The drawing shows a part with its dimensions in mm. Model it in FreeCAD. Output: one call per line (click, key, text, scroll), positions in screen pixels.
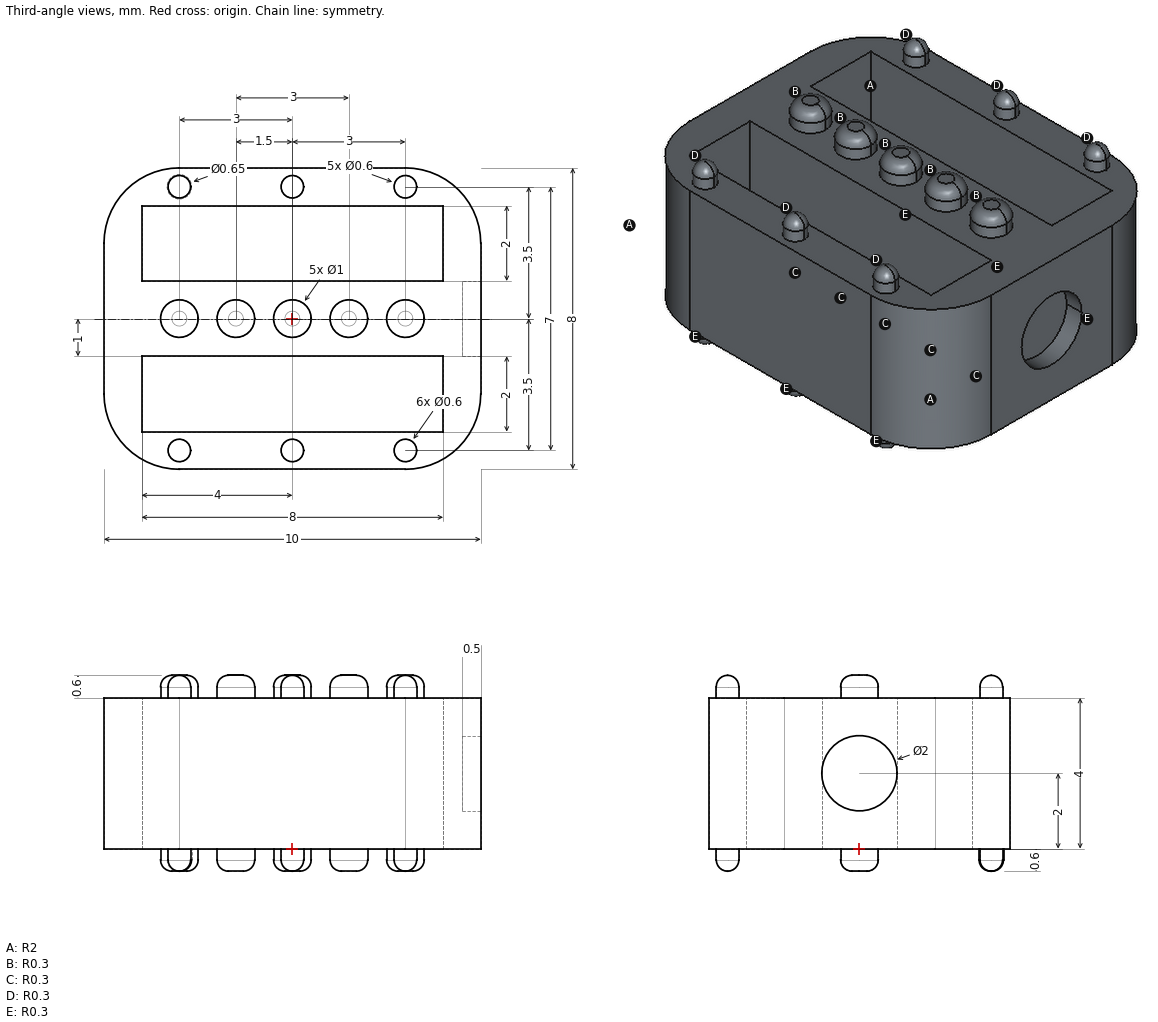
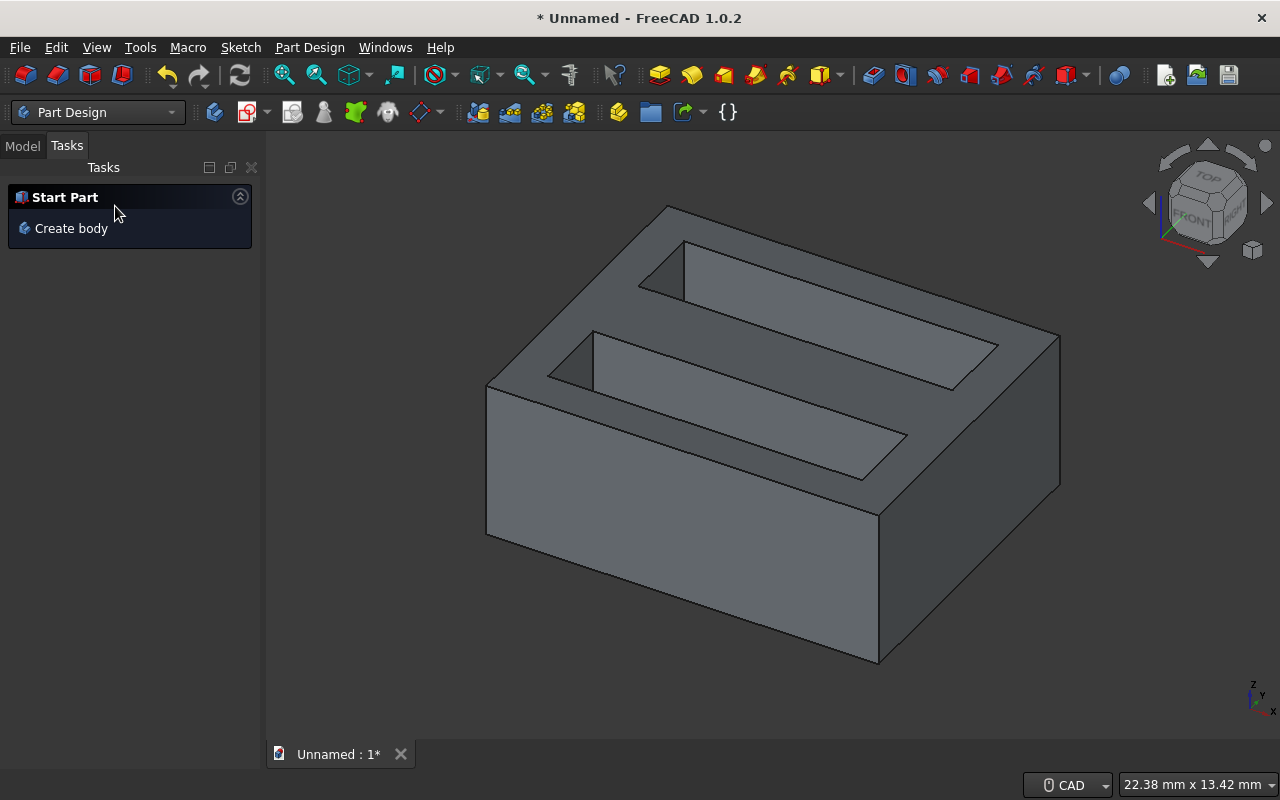
click(995, 473)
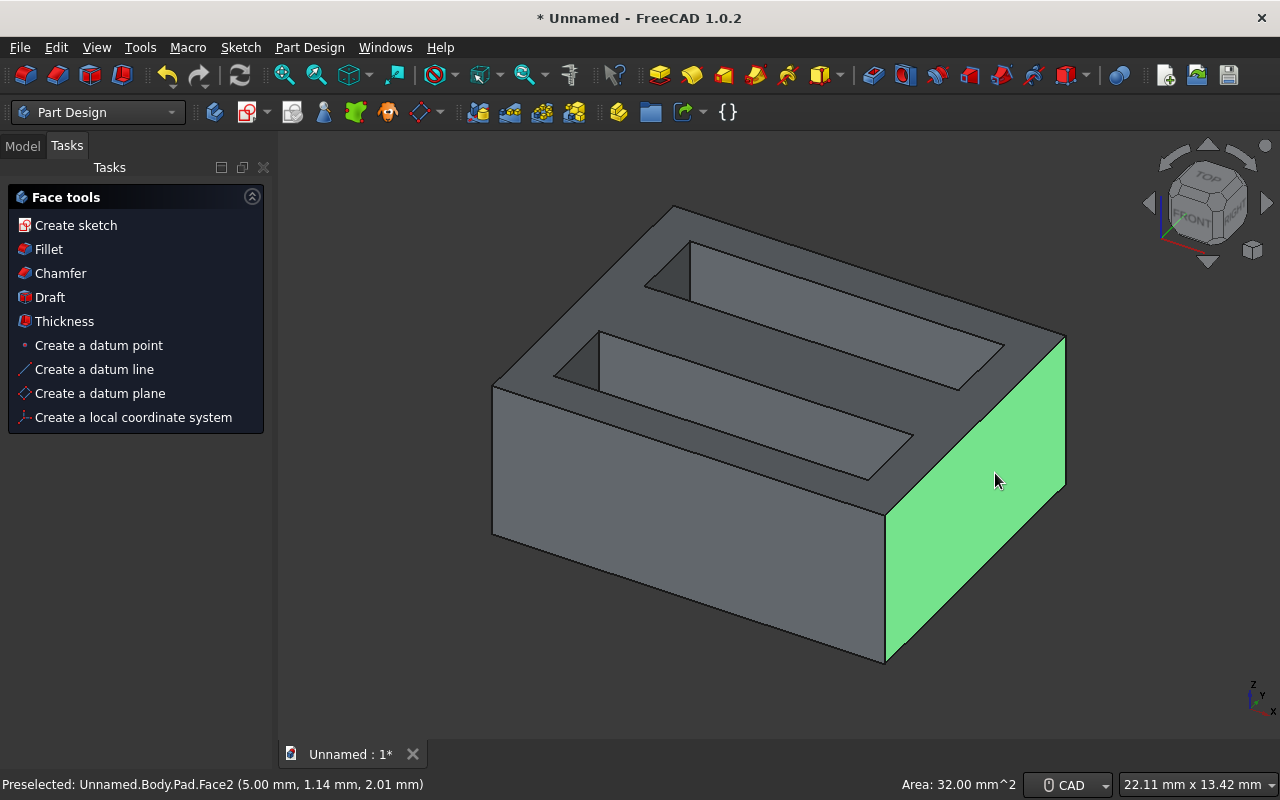
click(248, 112)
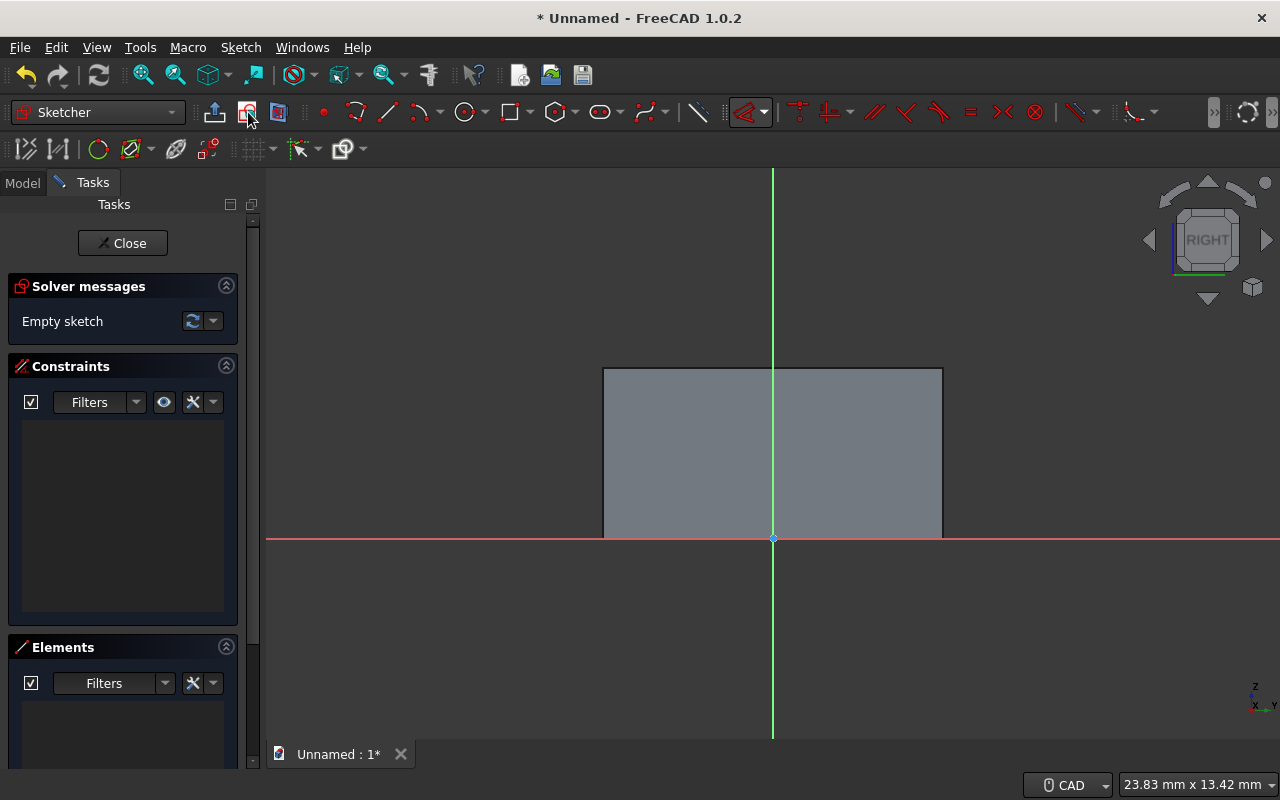
scroll(813, 487, up, 5)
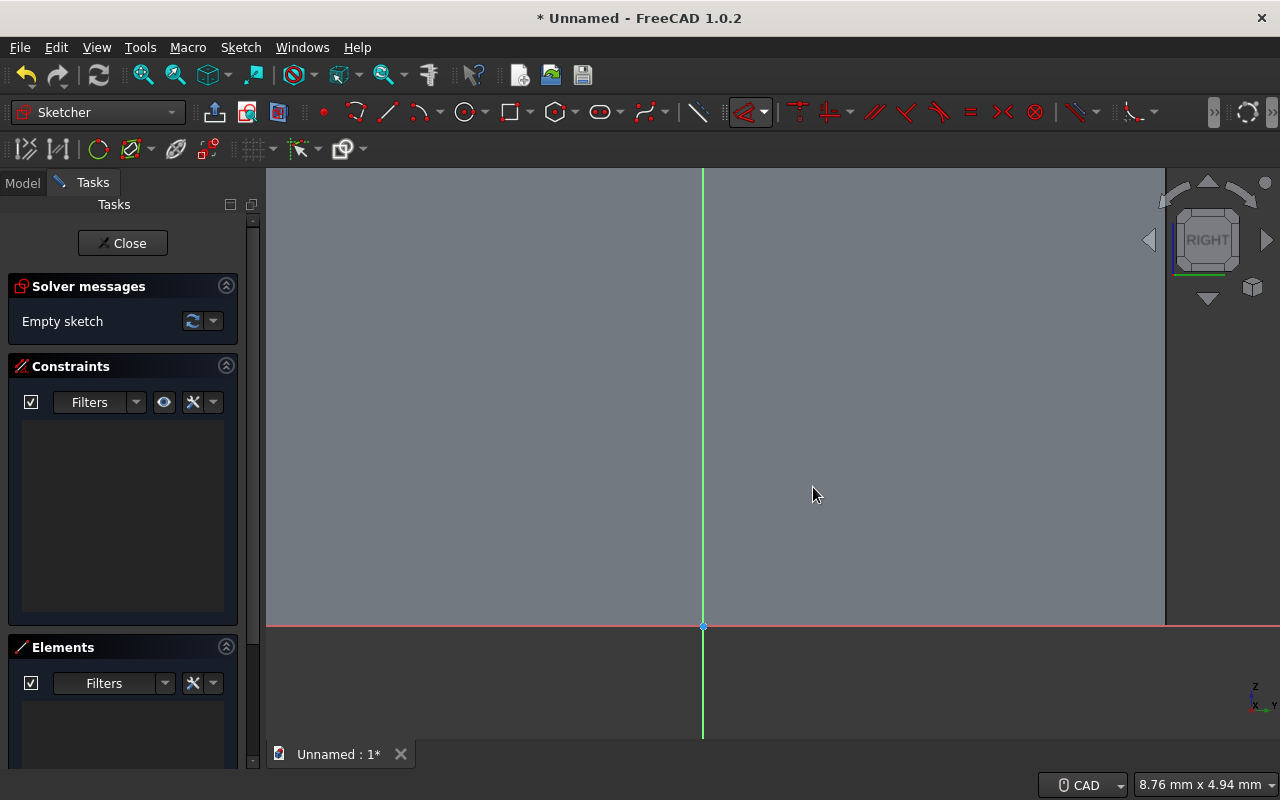
click(466, 112)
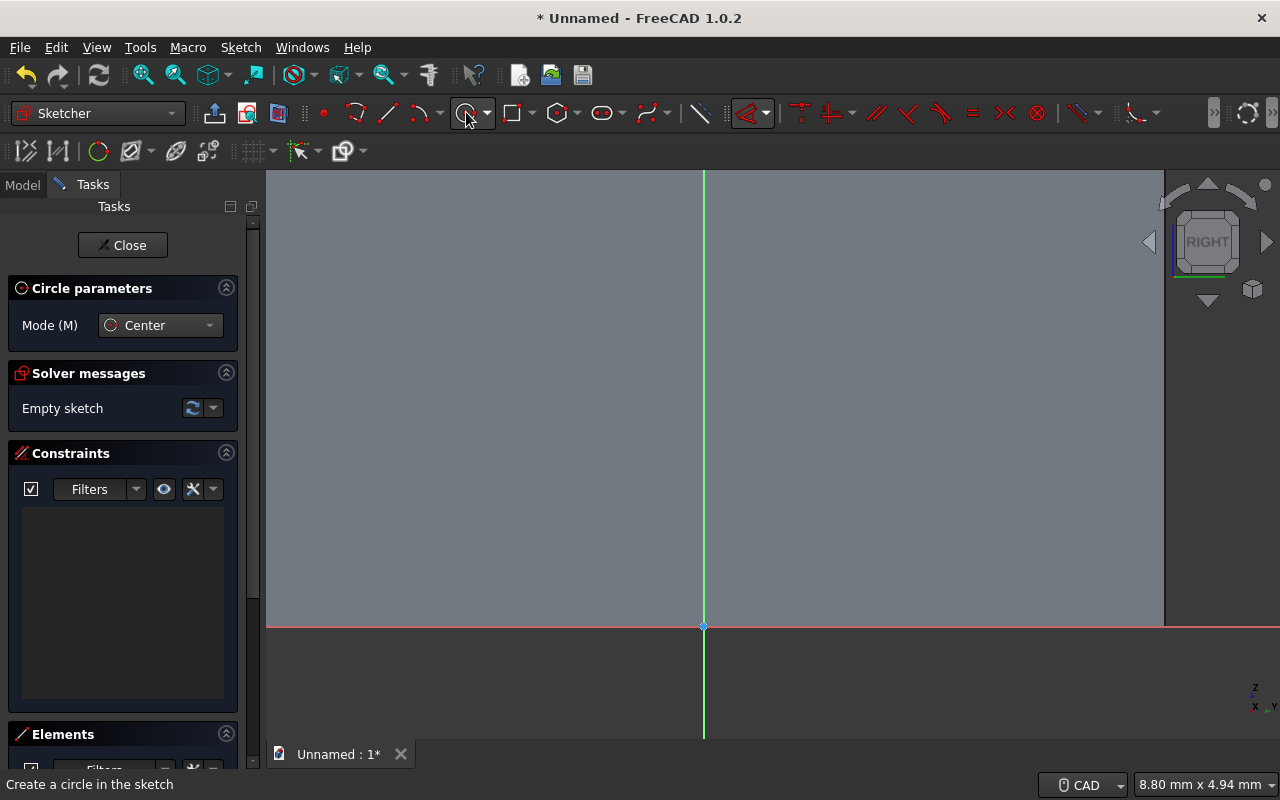
click(704, 396)
move(785, 315)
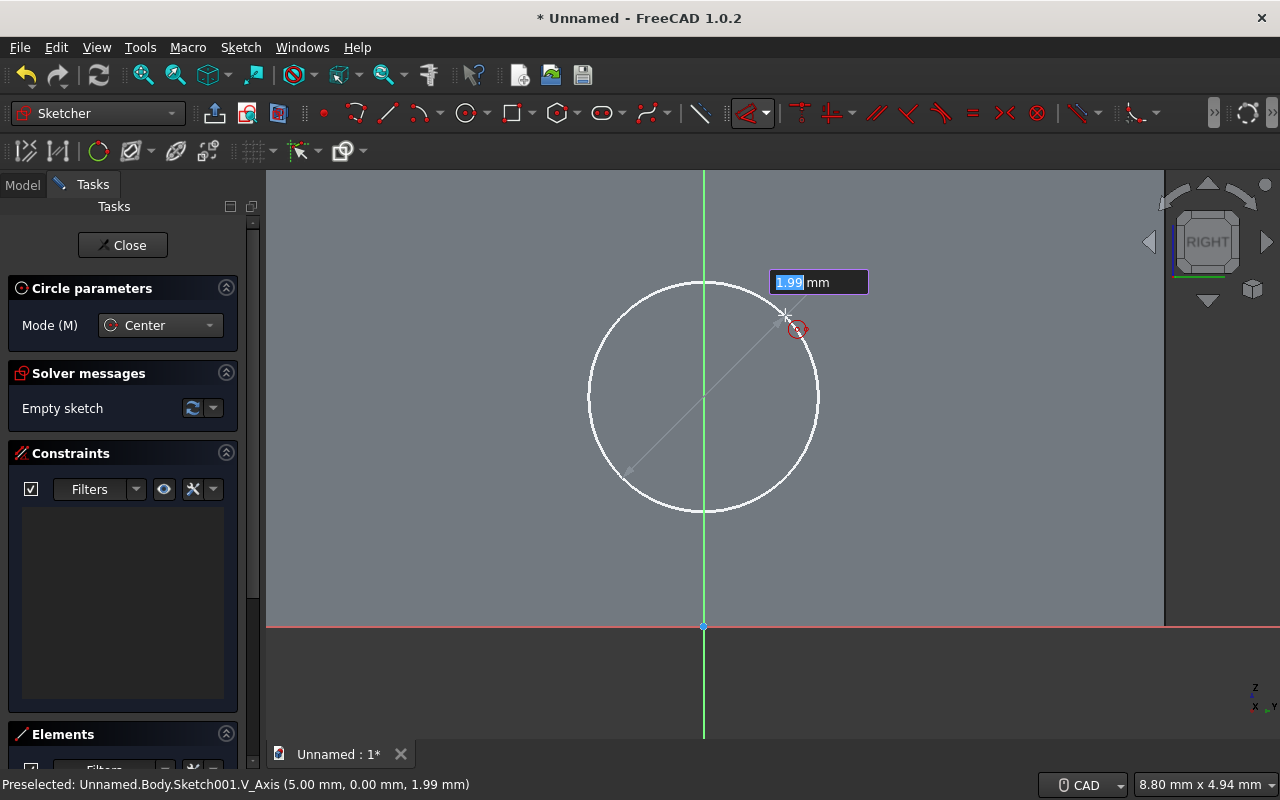
text(2)
key(Return)
key(Escape)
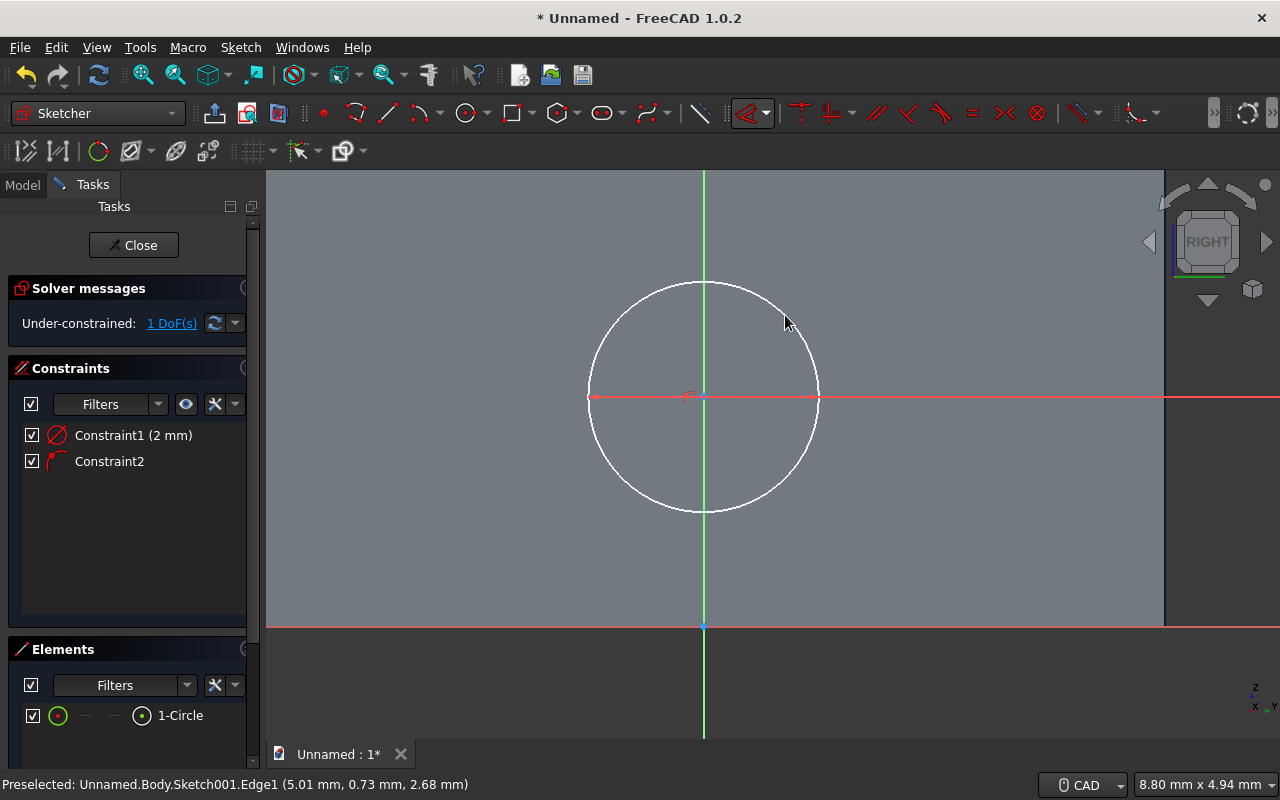
click(704, 397)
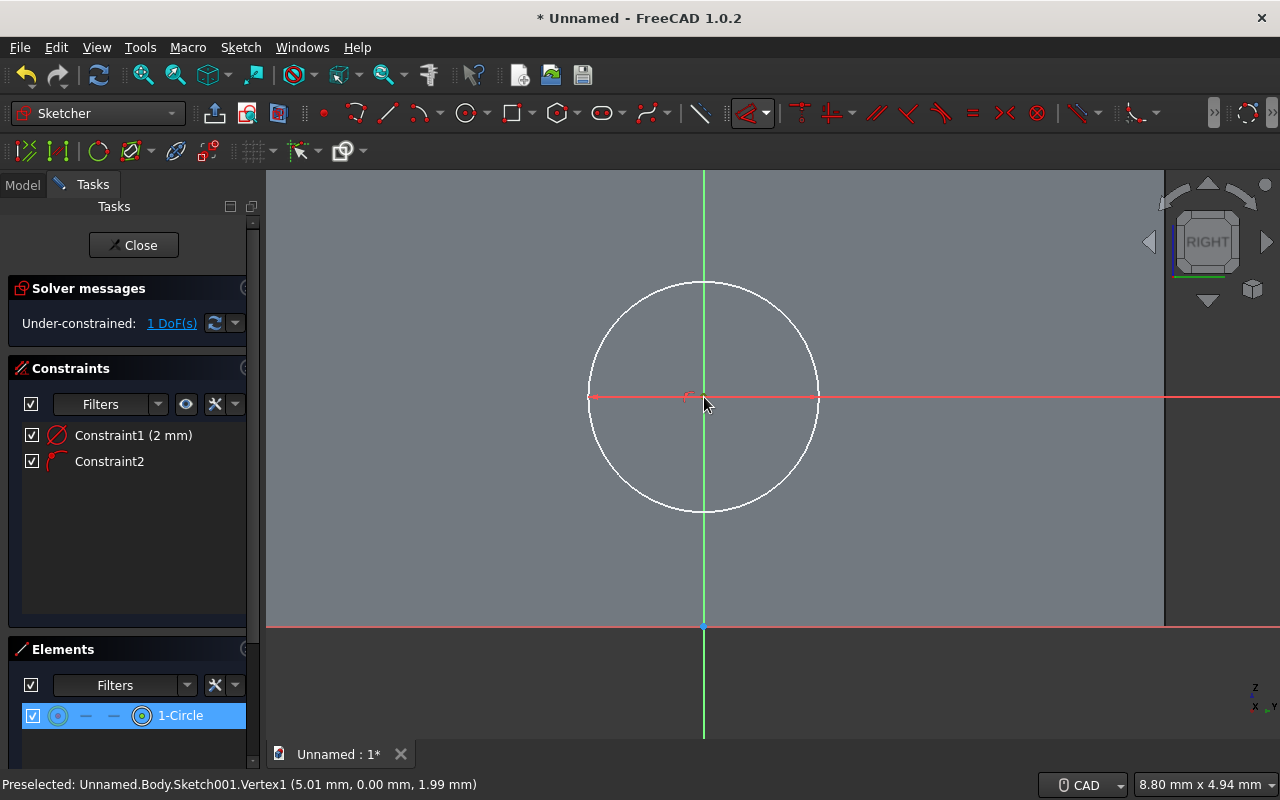
key(i)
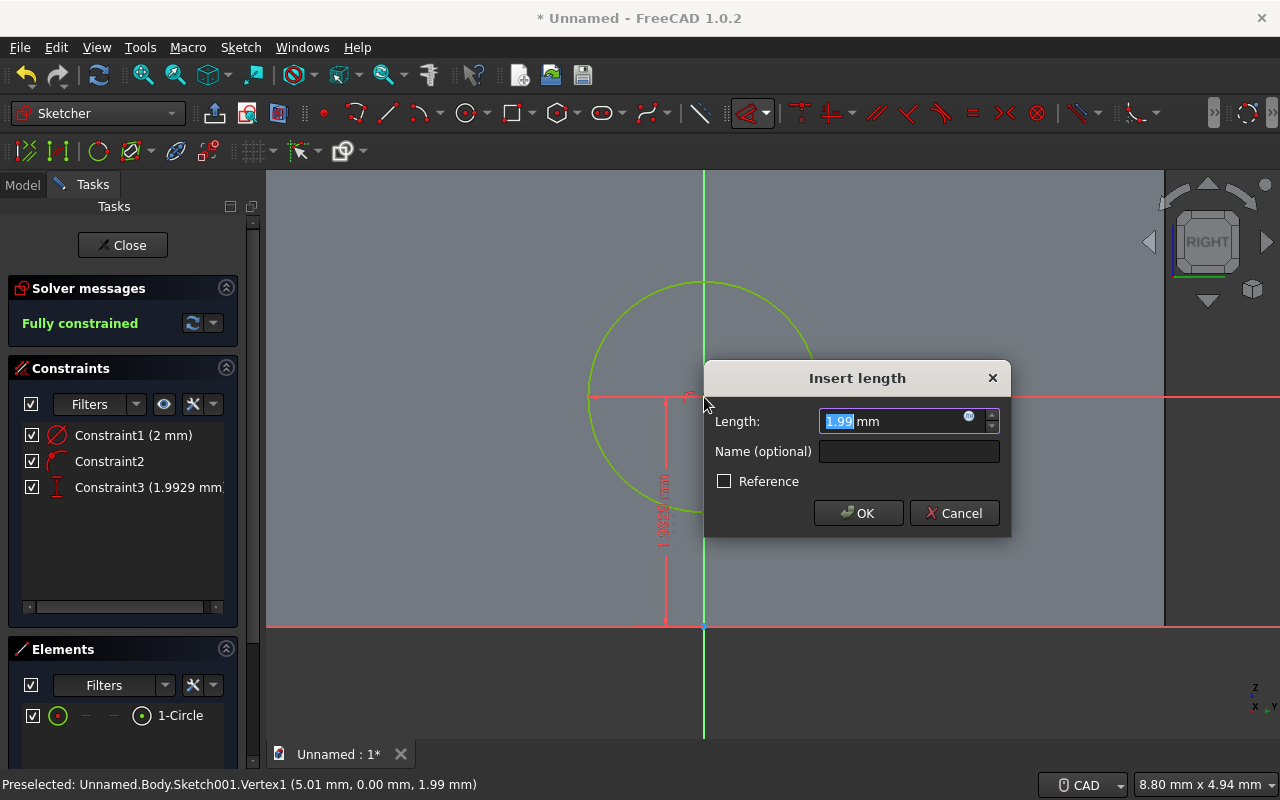
text(2)
key(Return)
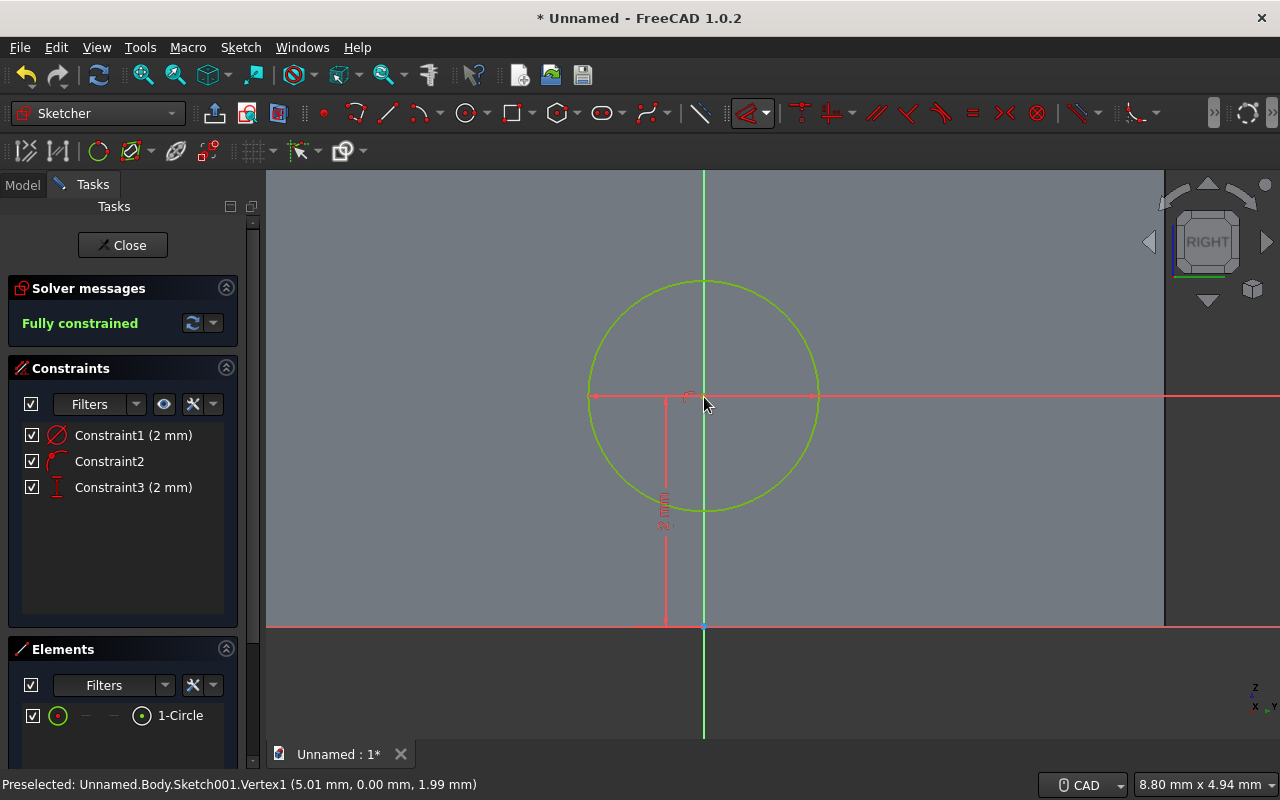
click(123, 245)